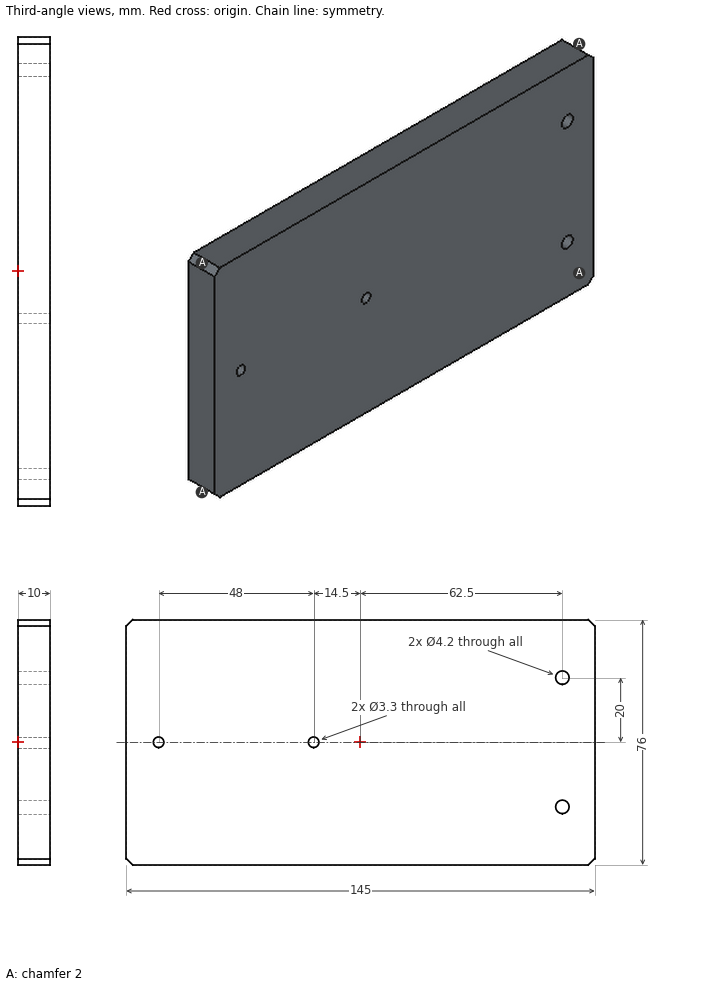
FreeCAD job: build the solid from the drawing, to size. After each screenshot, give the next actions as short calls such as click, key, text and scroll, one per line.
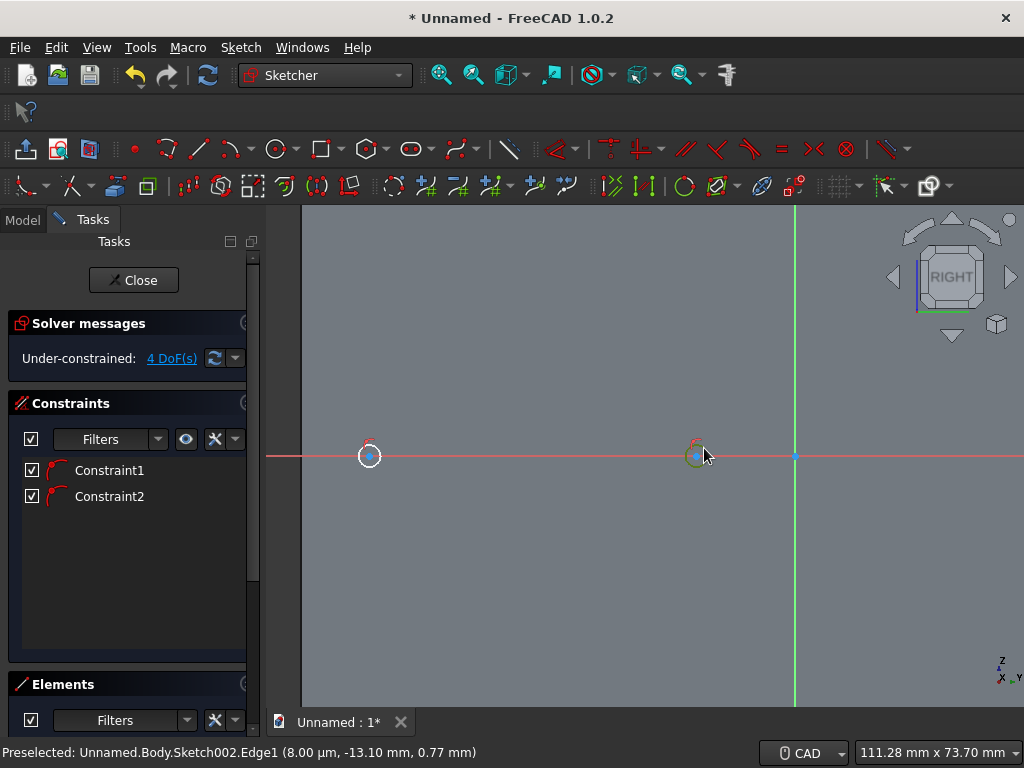
scroll(377, 448, up, 3)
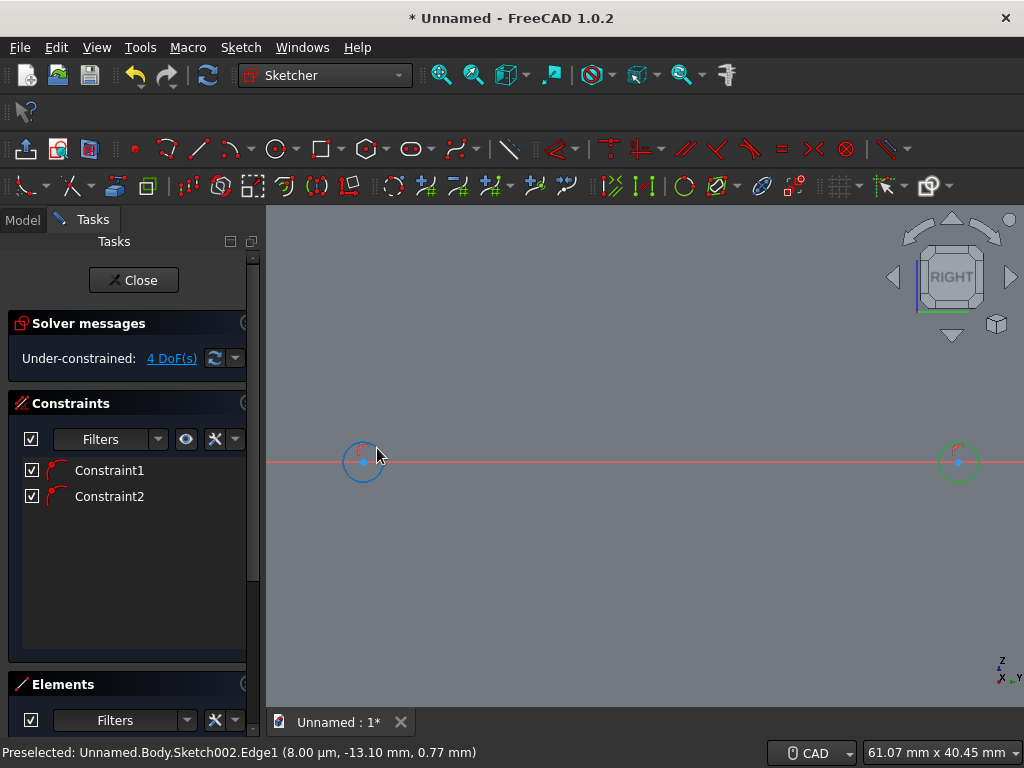
click(377, 448)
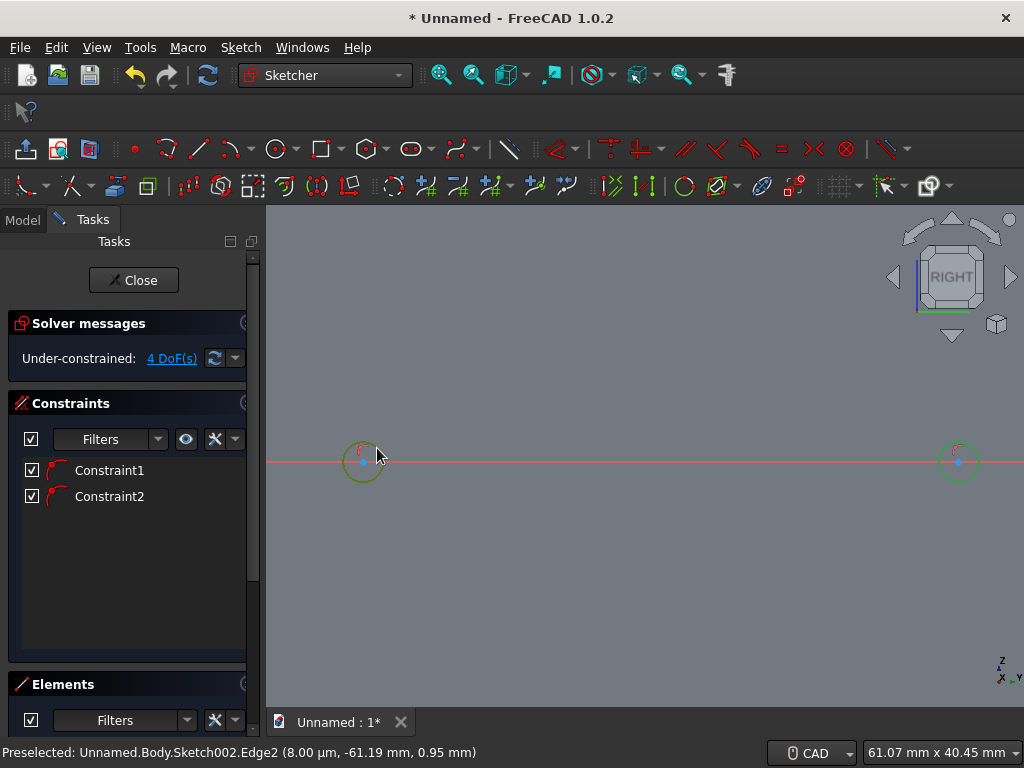
key(e)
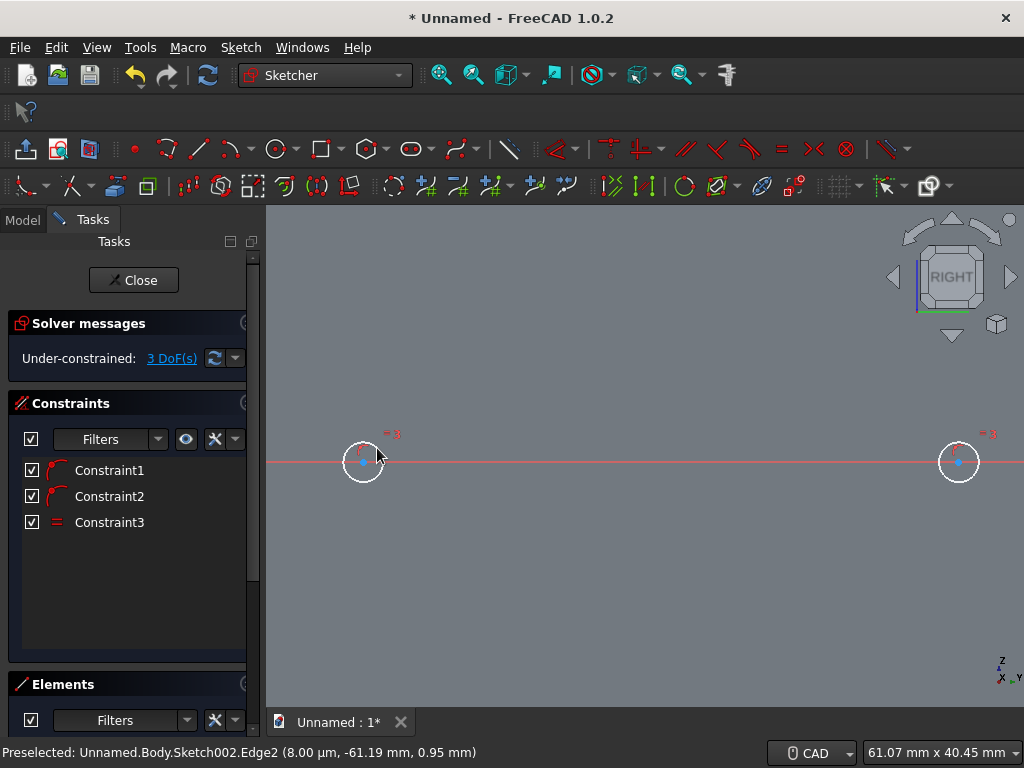
click(556, 150)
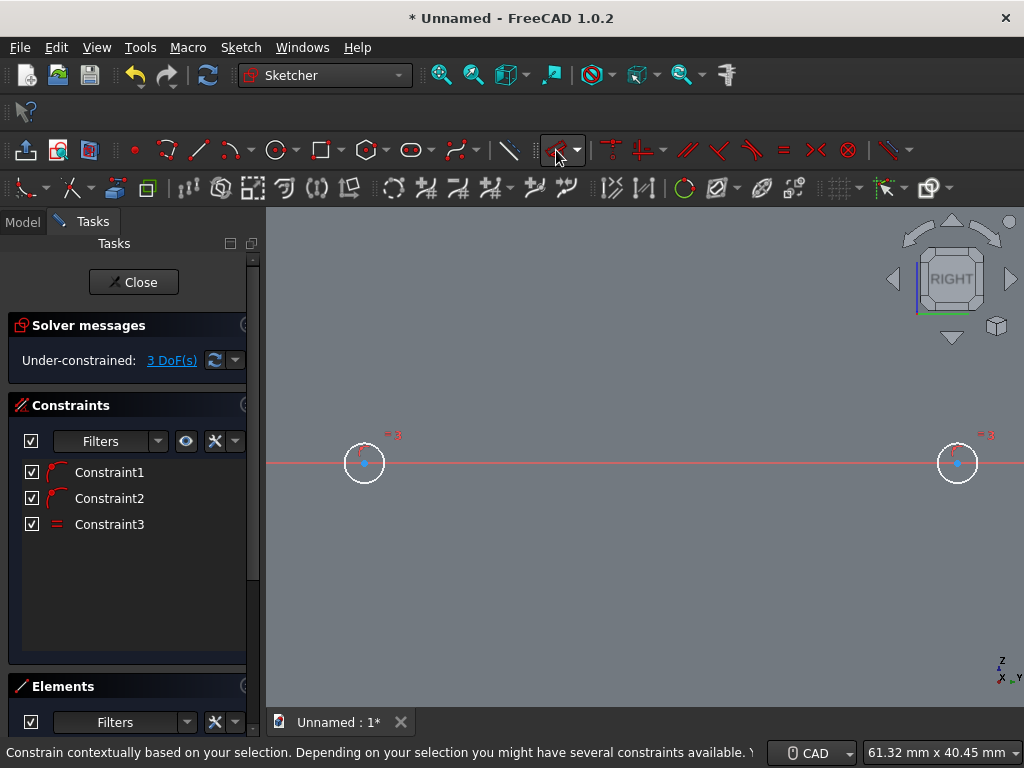
scroll(377, 449, down, 3)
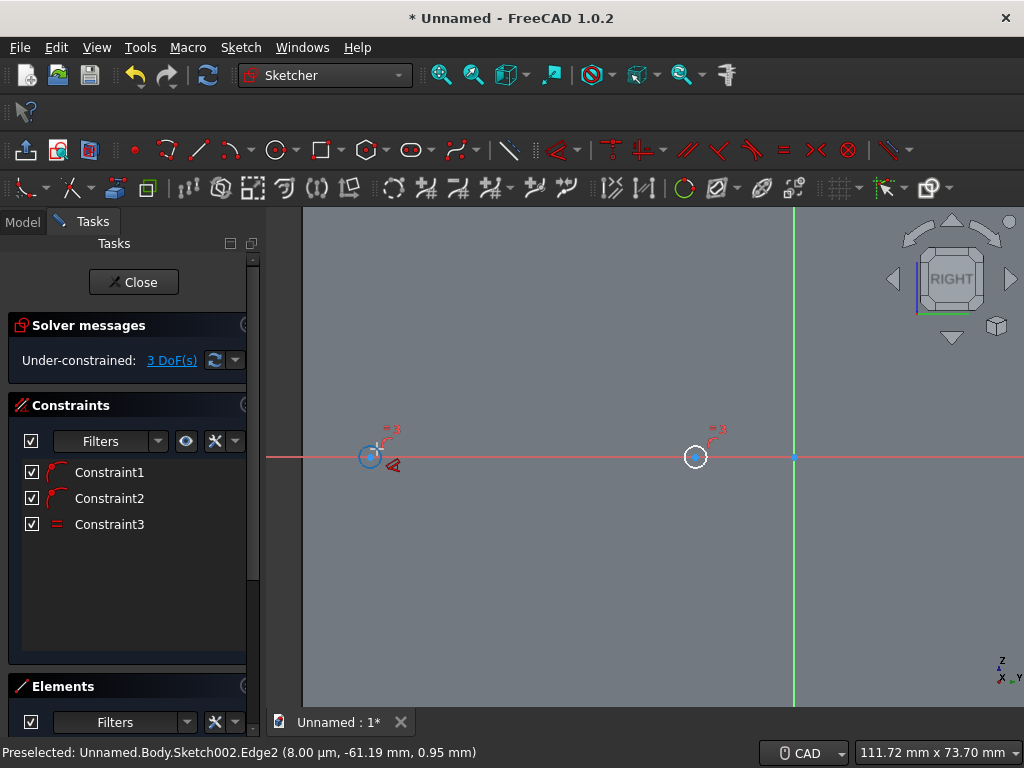
scroll(703, 449, up, 3)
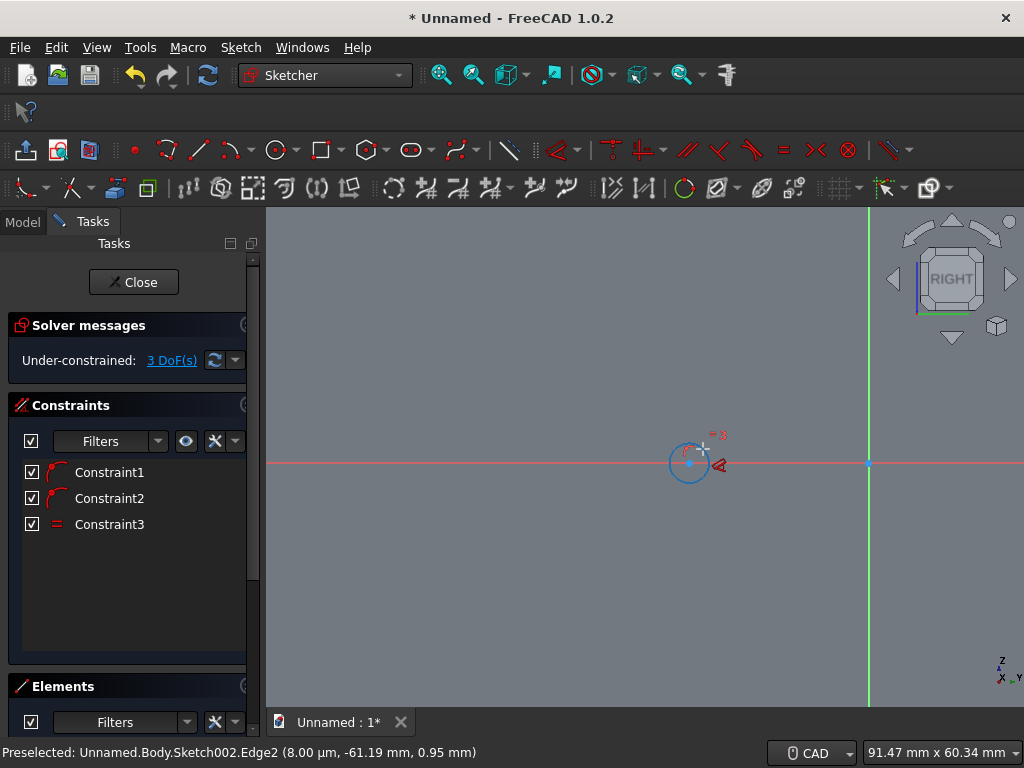
click(703, 449)
click(725, 426)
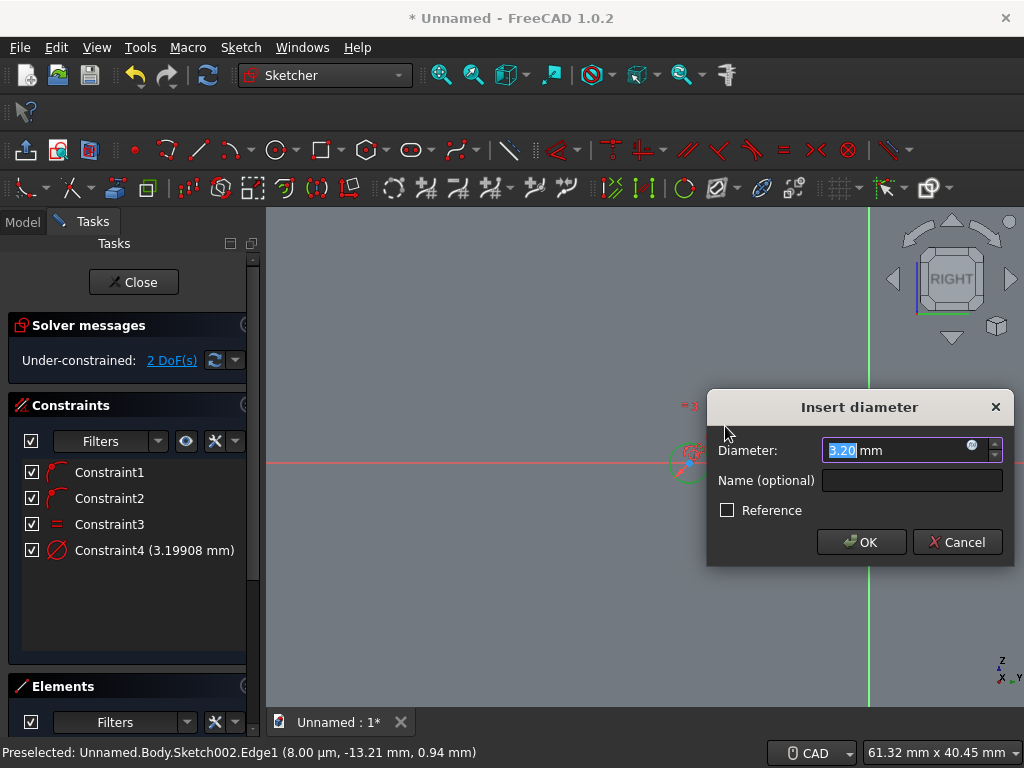
text(3.3)
key(Return)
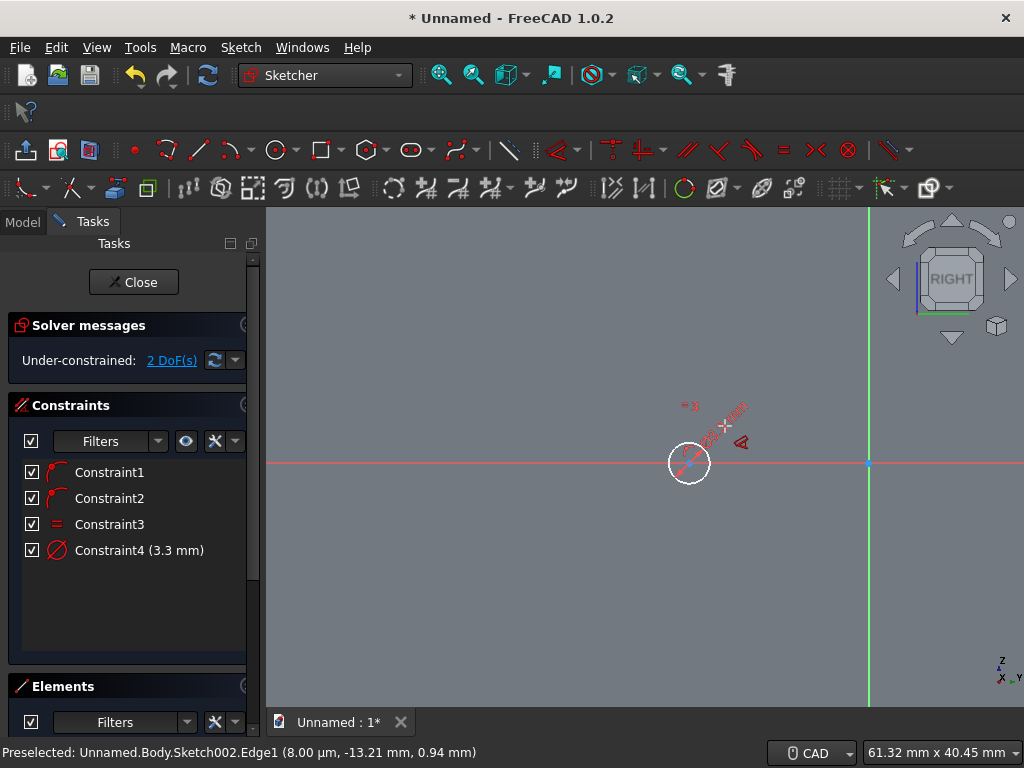
click(689, 463)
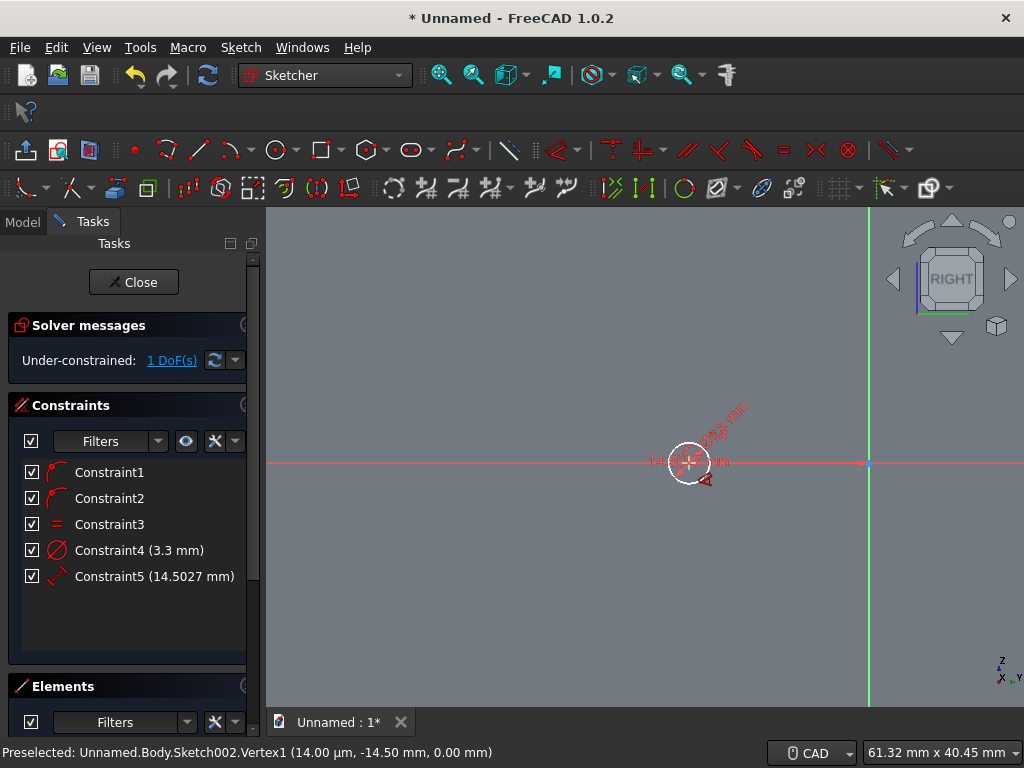
scroll(704, 449, down, 3)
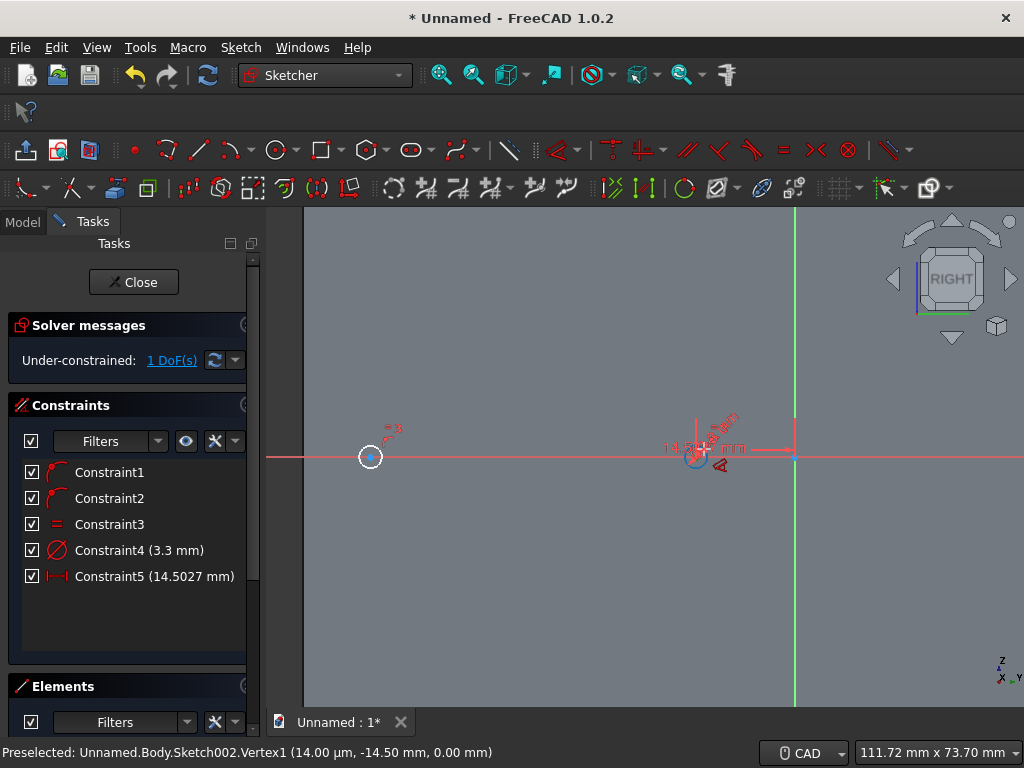
click(371, 457)
click(533, 491)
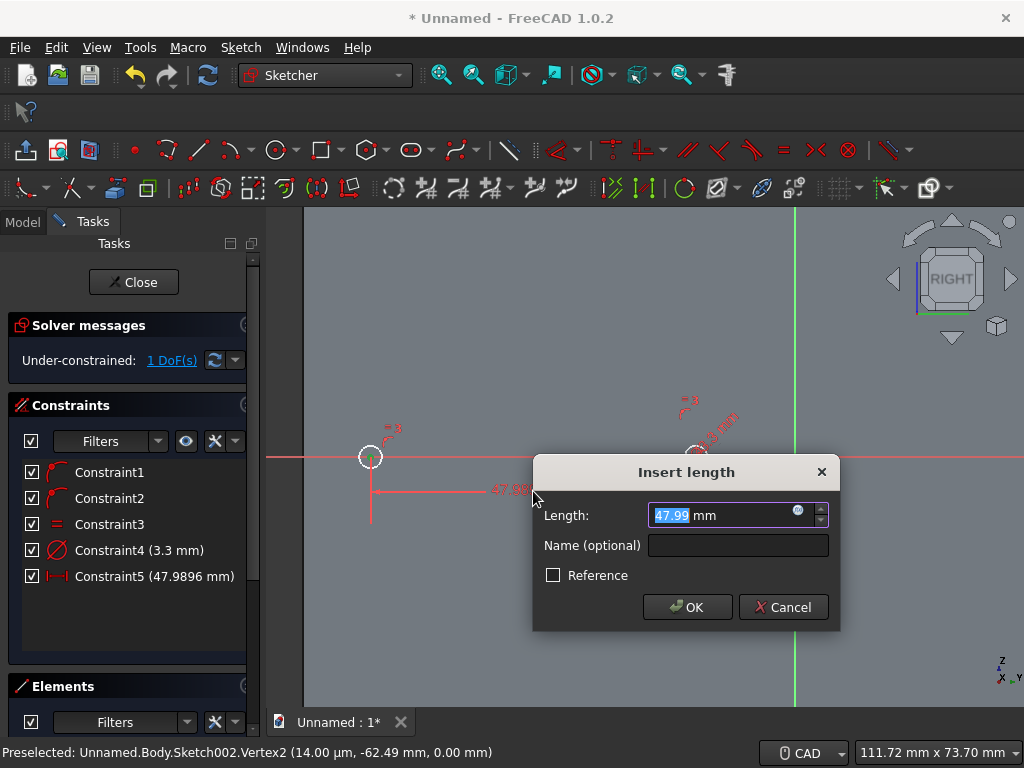
text(48)
key(Return)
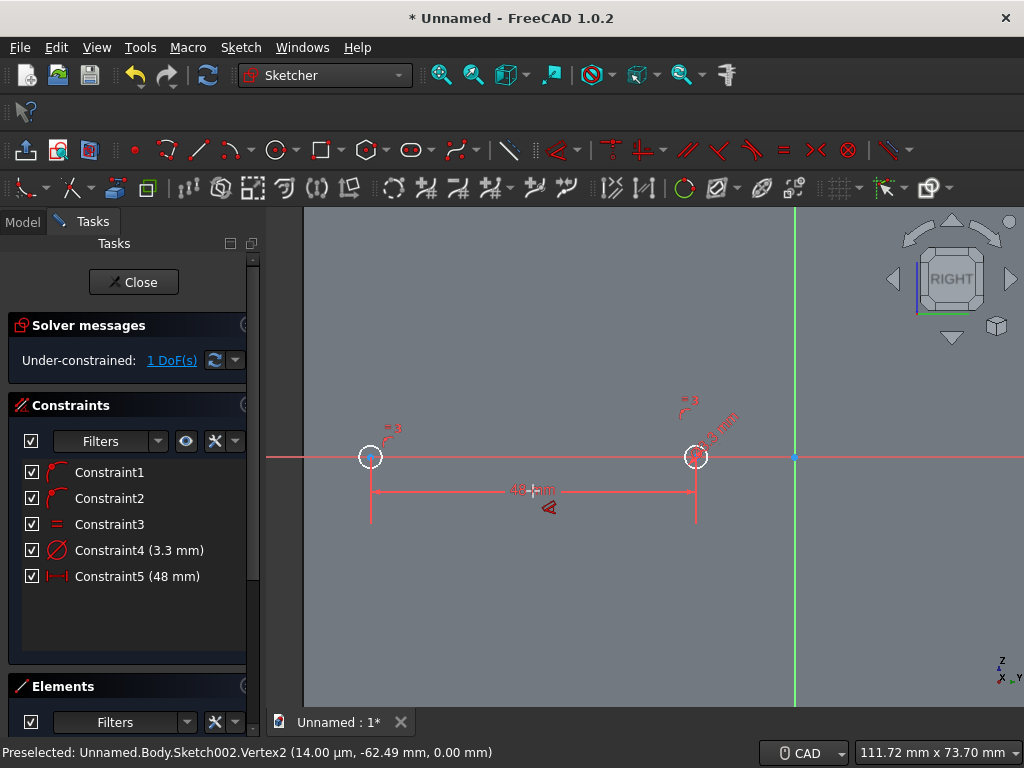
click(696, 457)
click(745, 491)